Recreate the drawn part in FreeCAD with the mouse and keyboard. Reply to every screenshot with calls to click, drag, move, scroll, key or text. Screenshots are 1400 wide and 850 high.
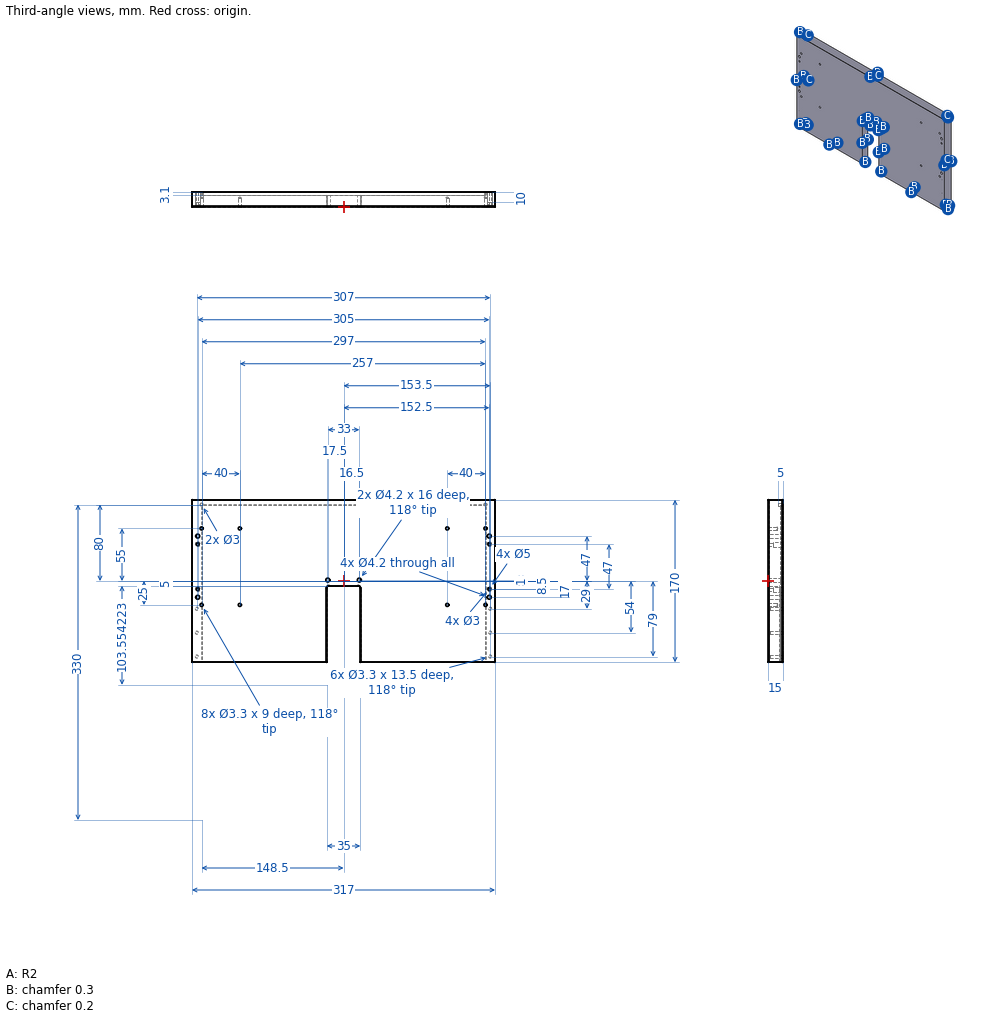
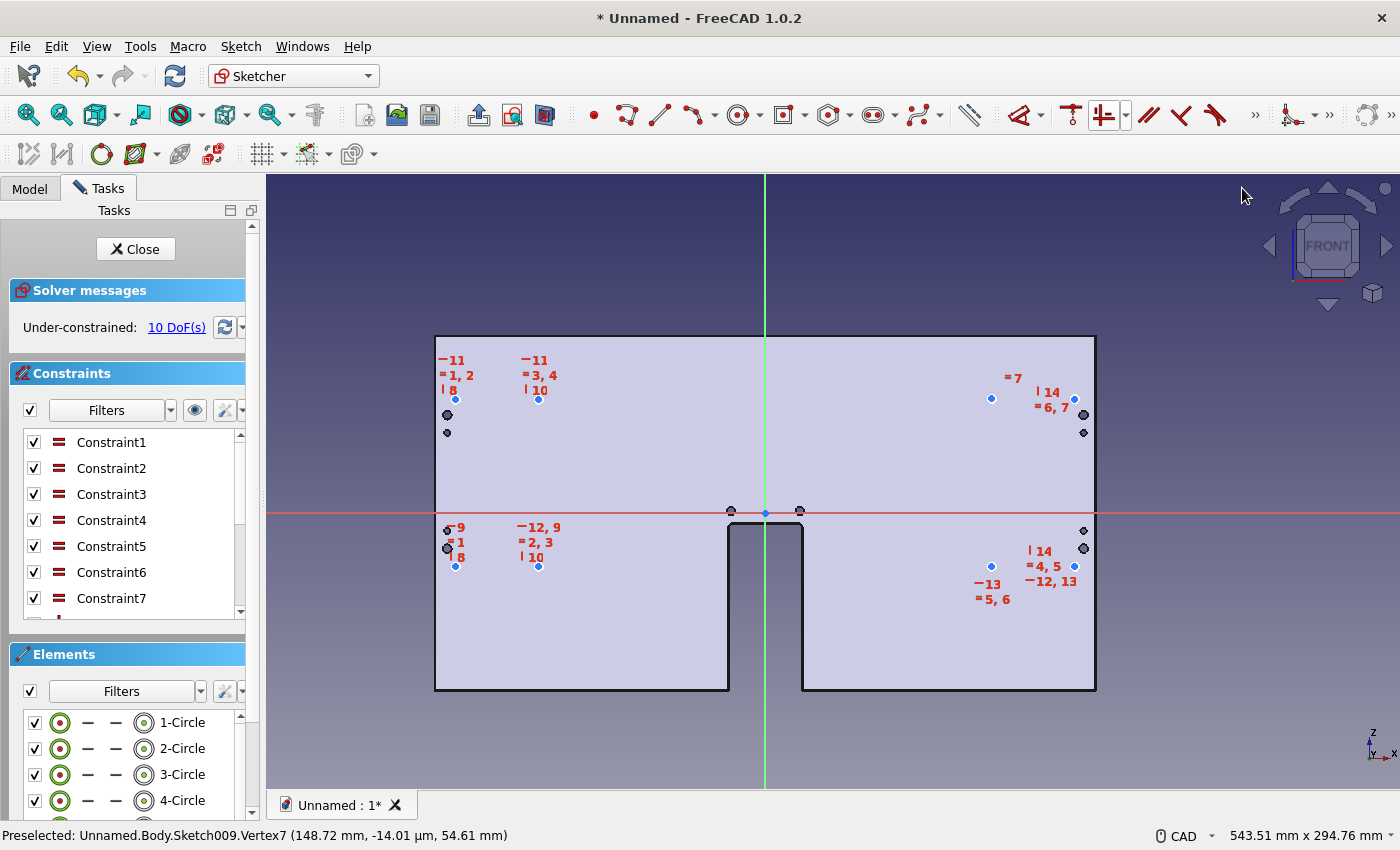
click(539, 400)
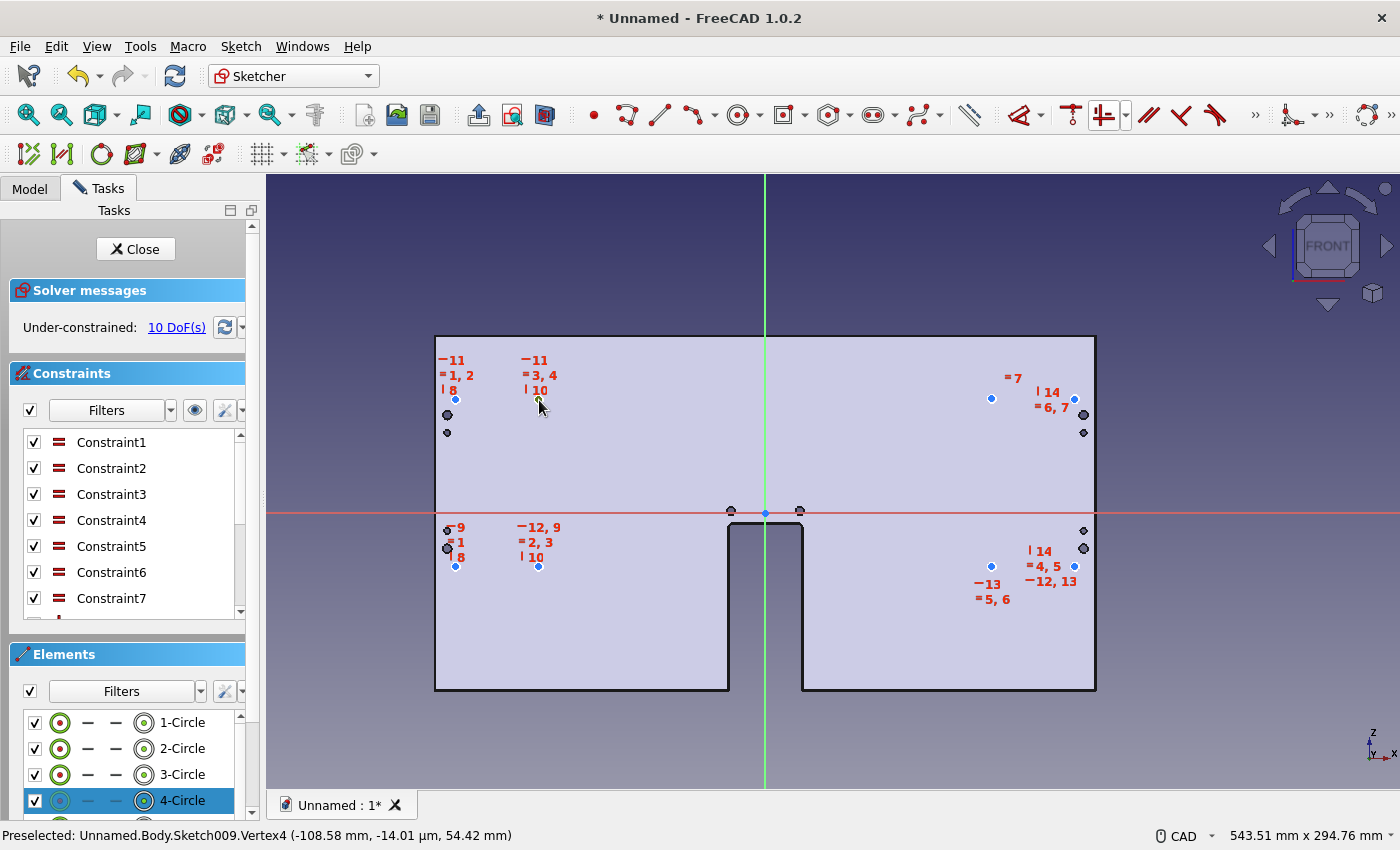
click(1075, 399)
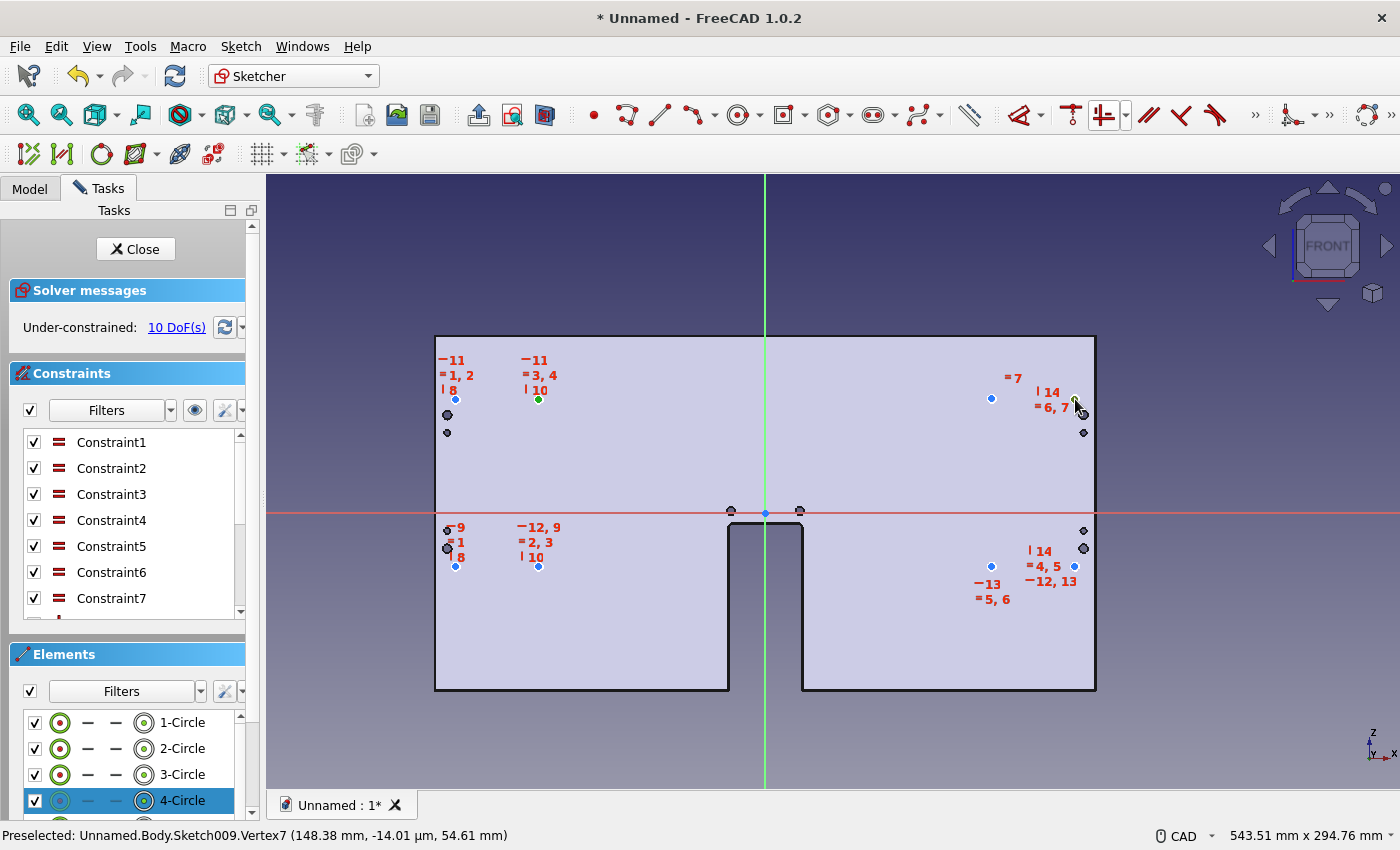
key(h)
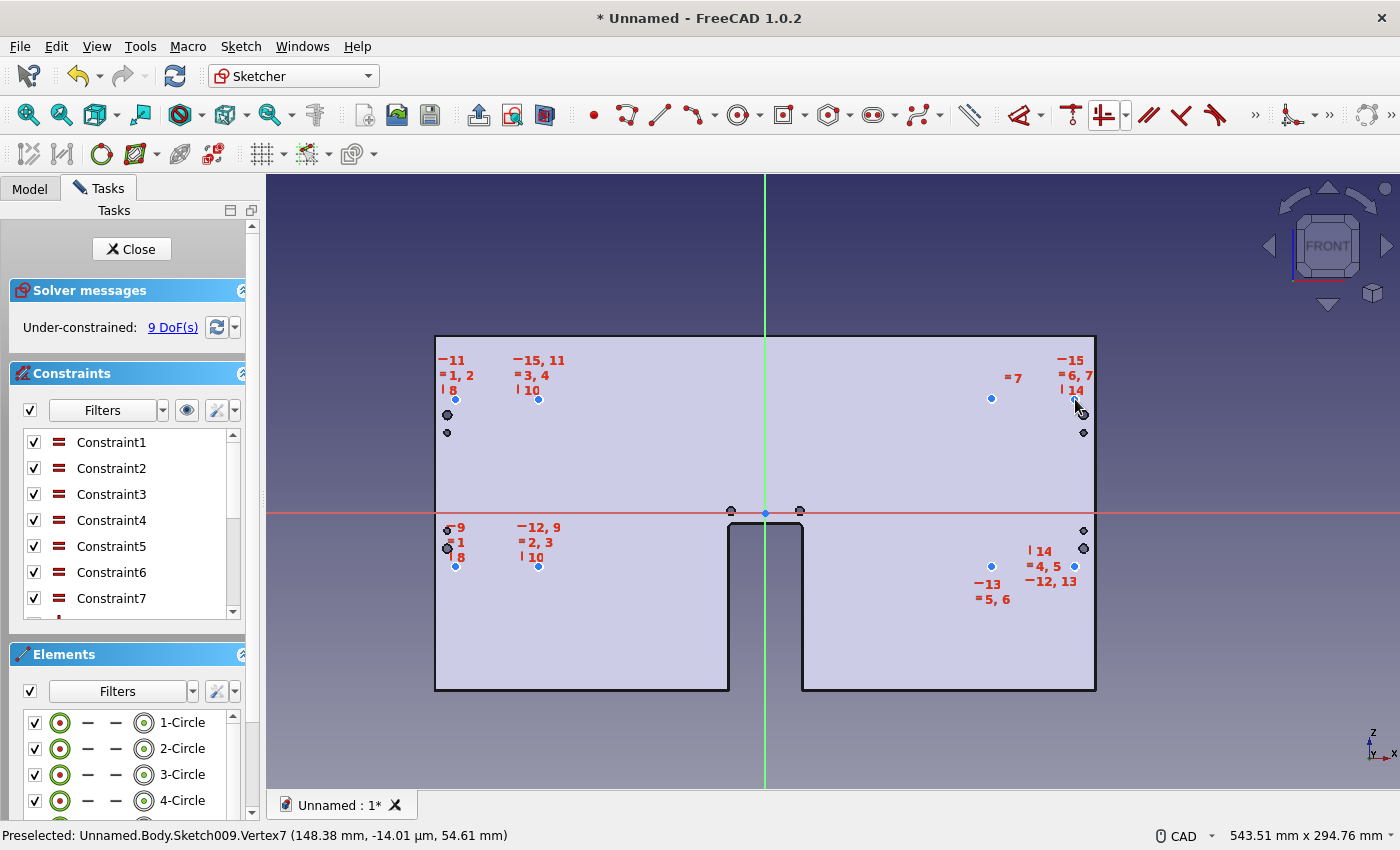
click(992, 567)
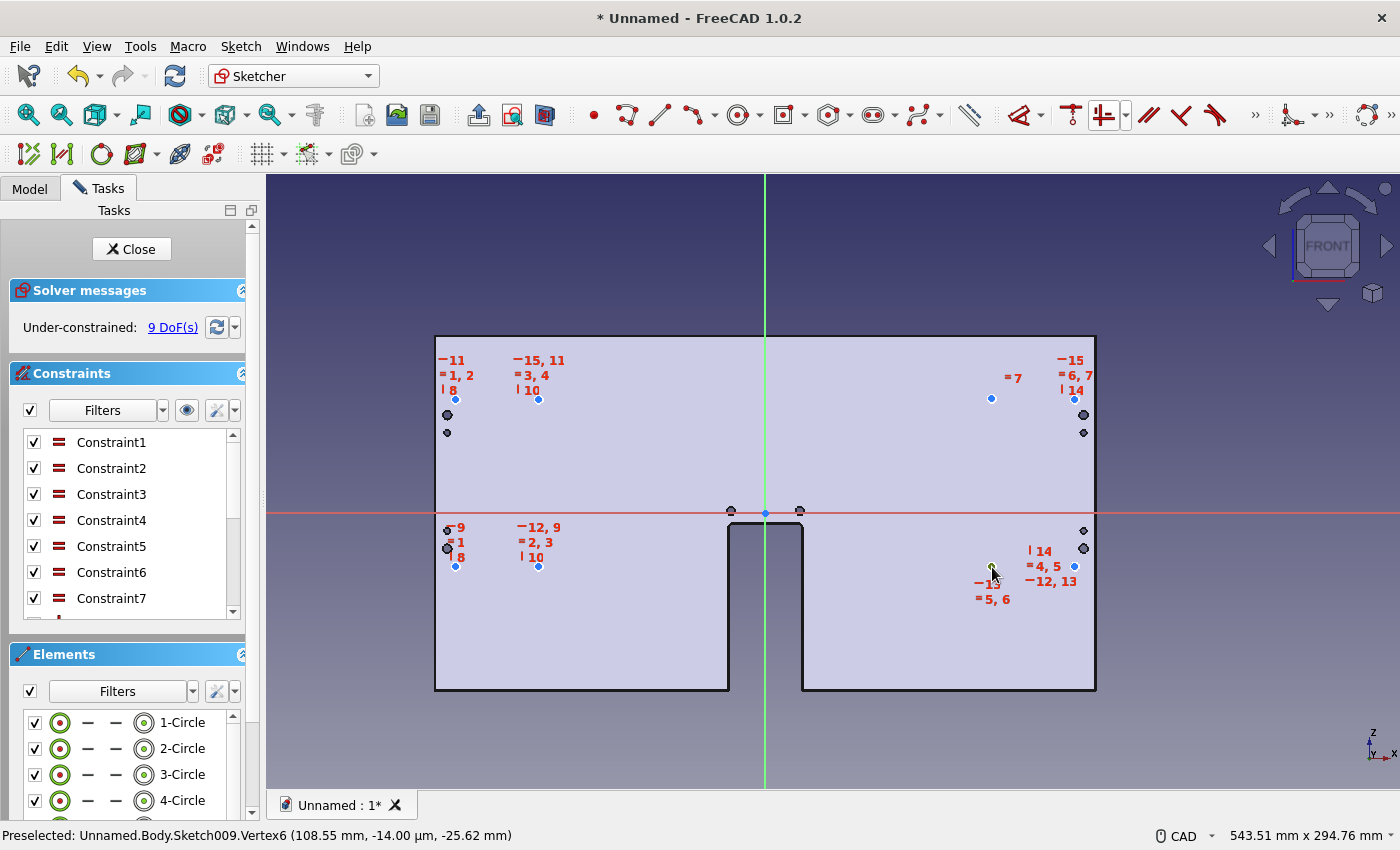
click(992, 399)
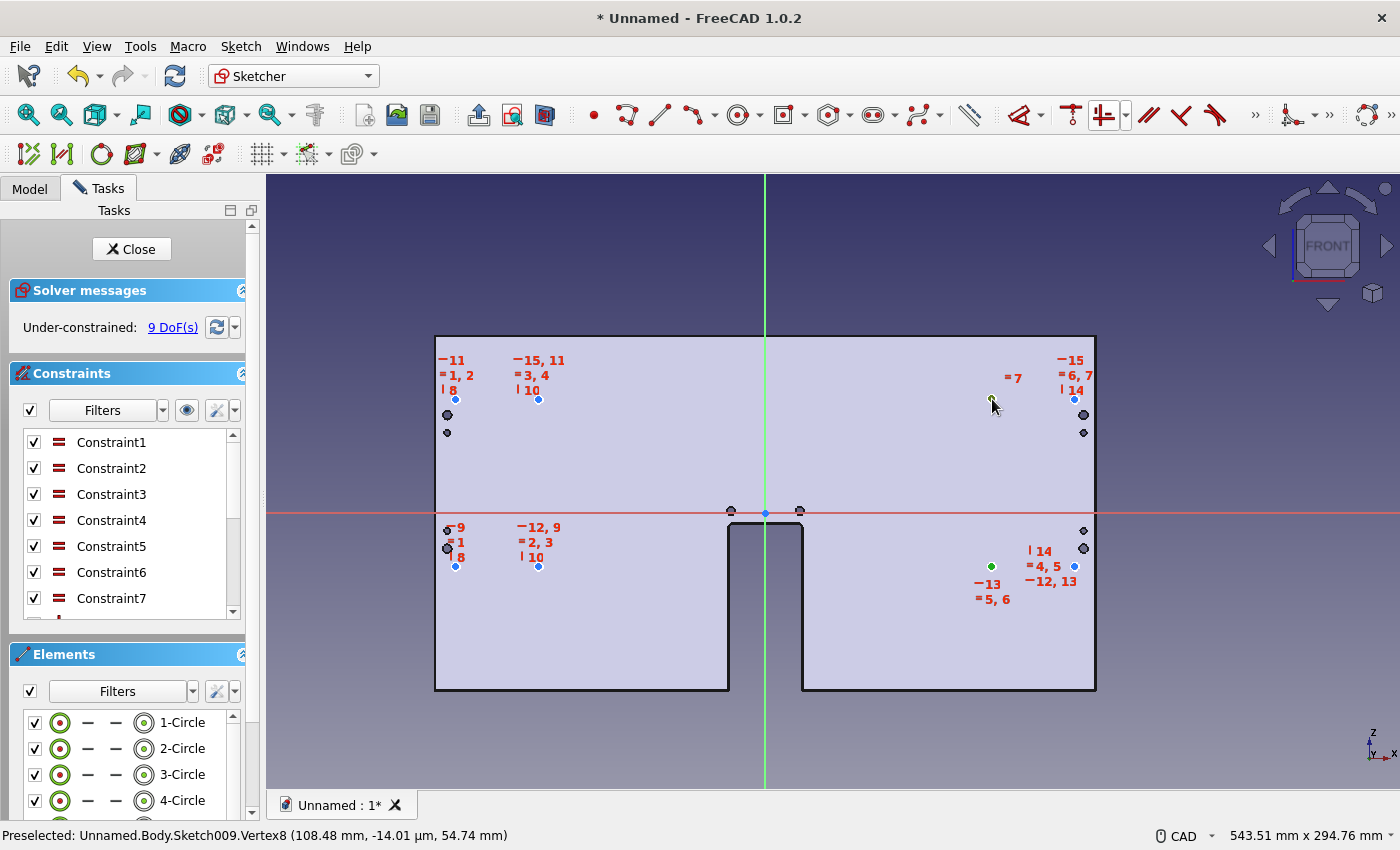
key(v)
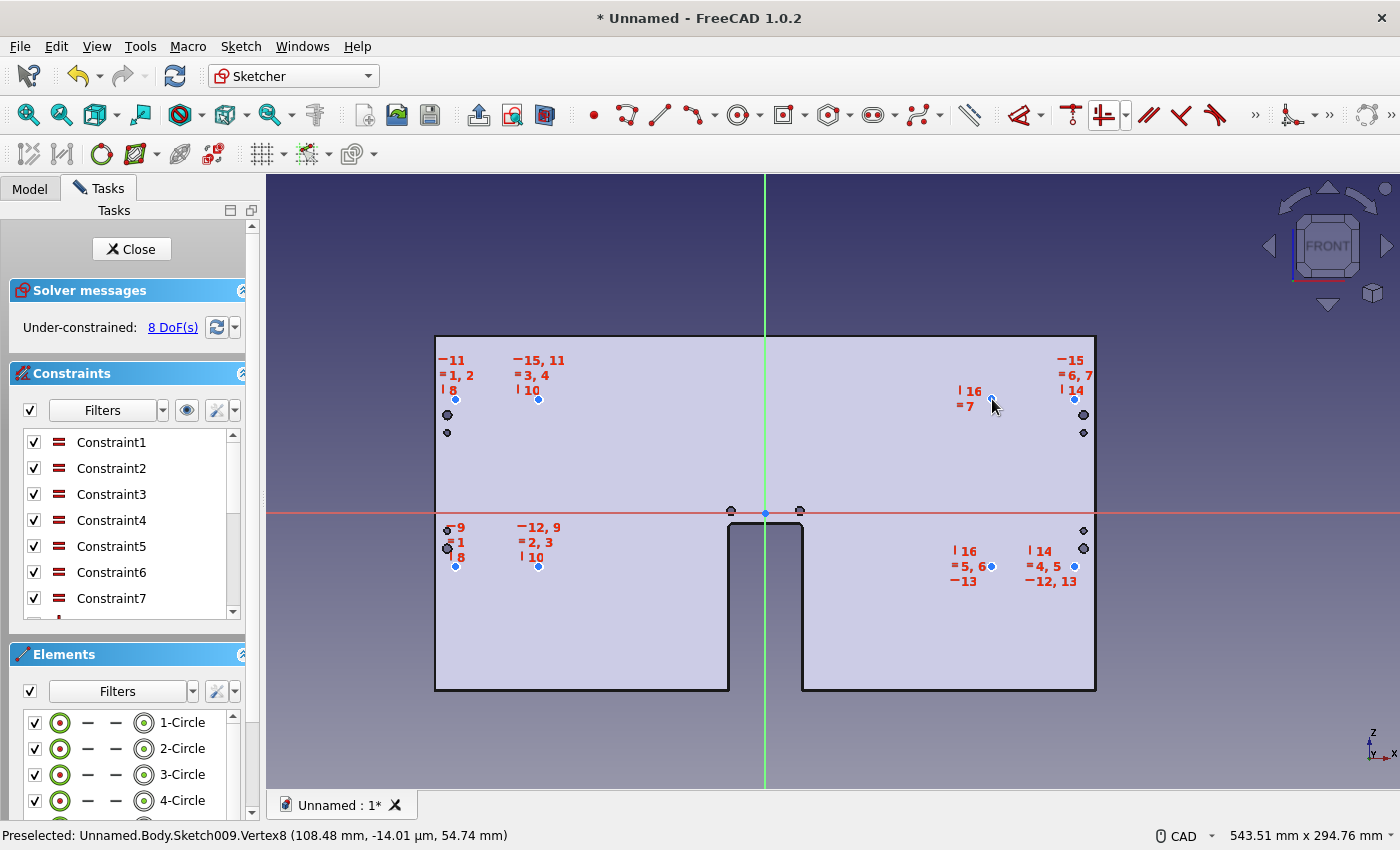
click(1075, 400)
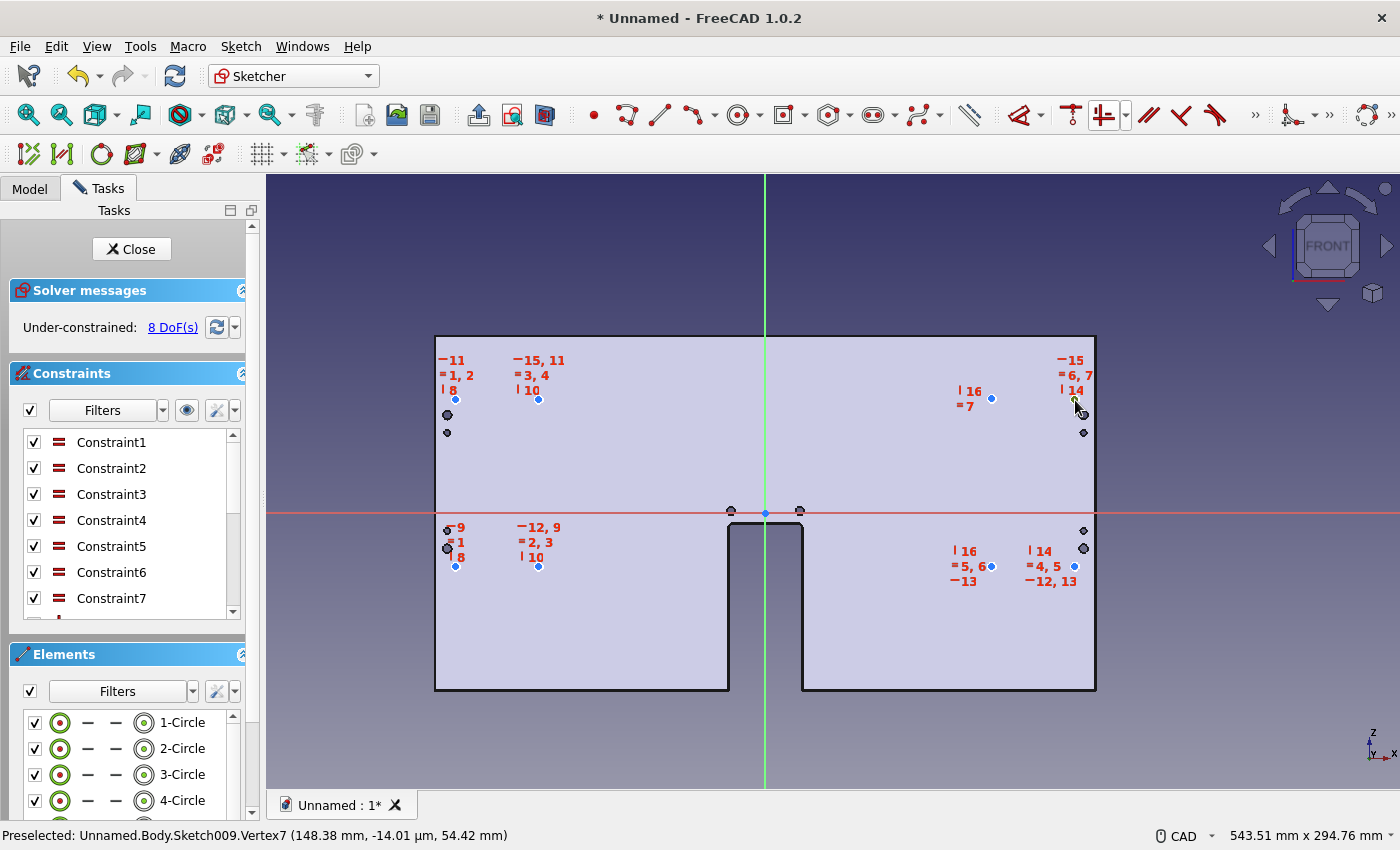
click(992, 399)